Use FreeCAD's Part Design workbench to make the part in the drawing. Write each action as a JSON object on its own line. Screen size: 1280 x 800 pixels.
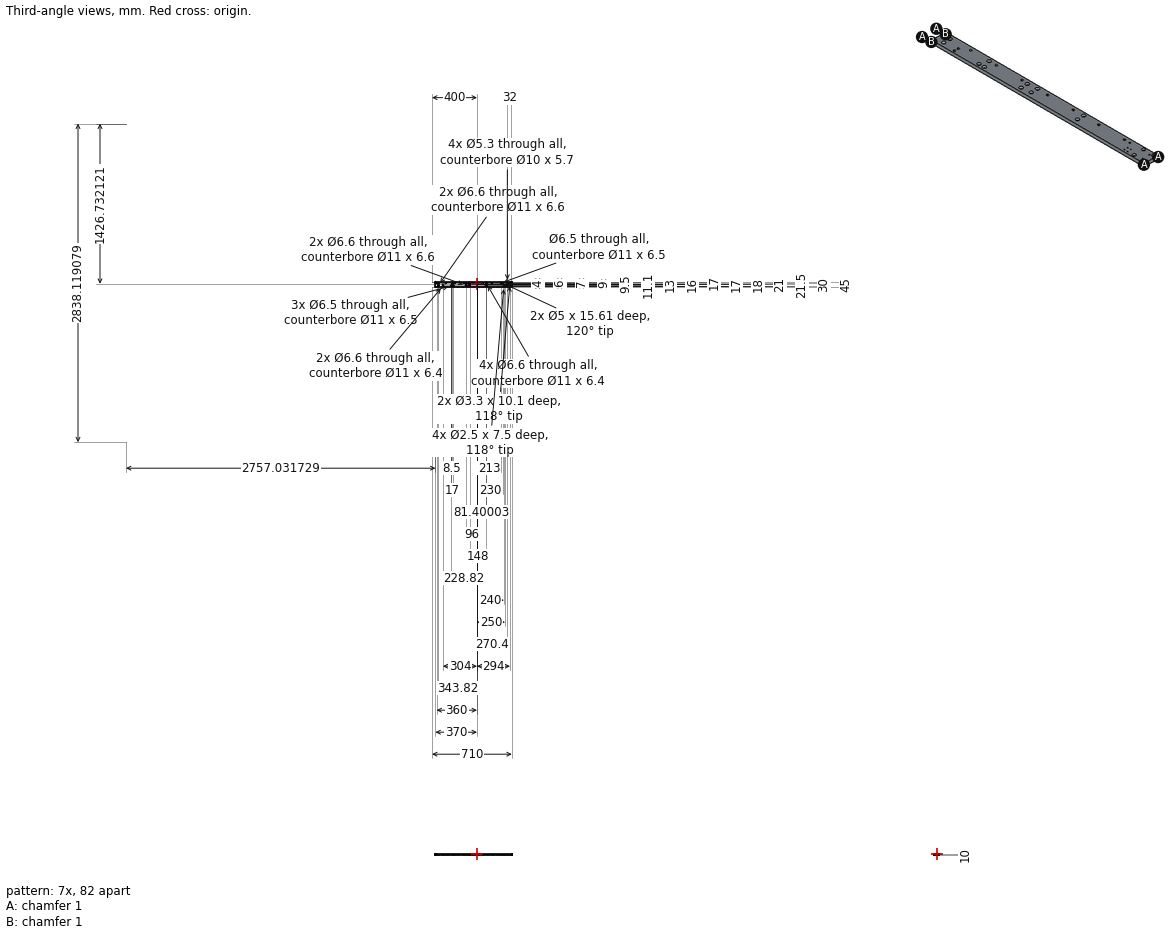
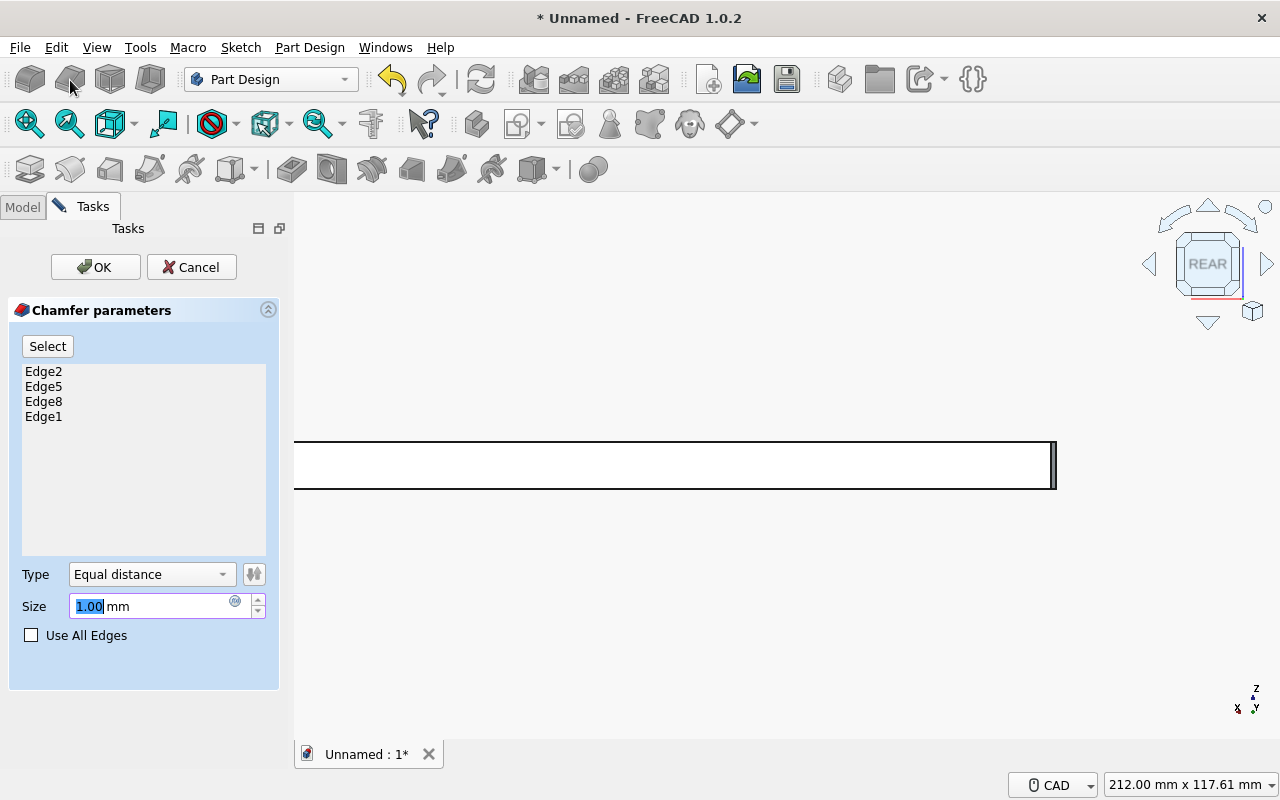
{"action": "type", "text": "1"}
{"action": "key", "text": "Tab"}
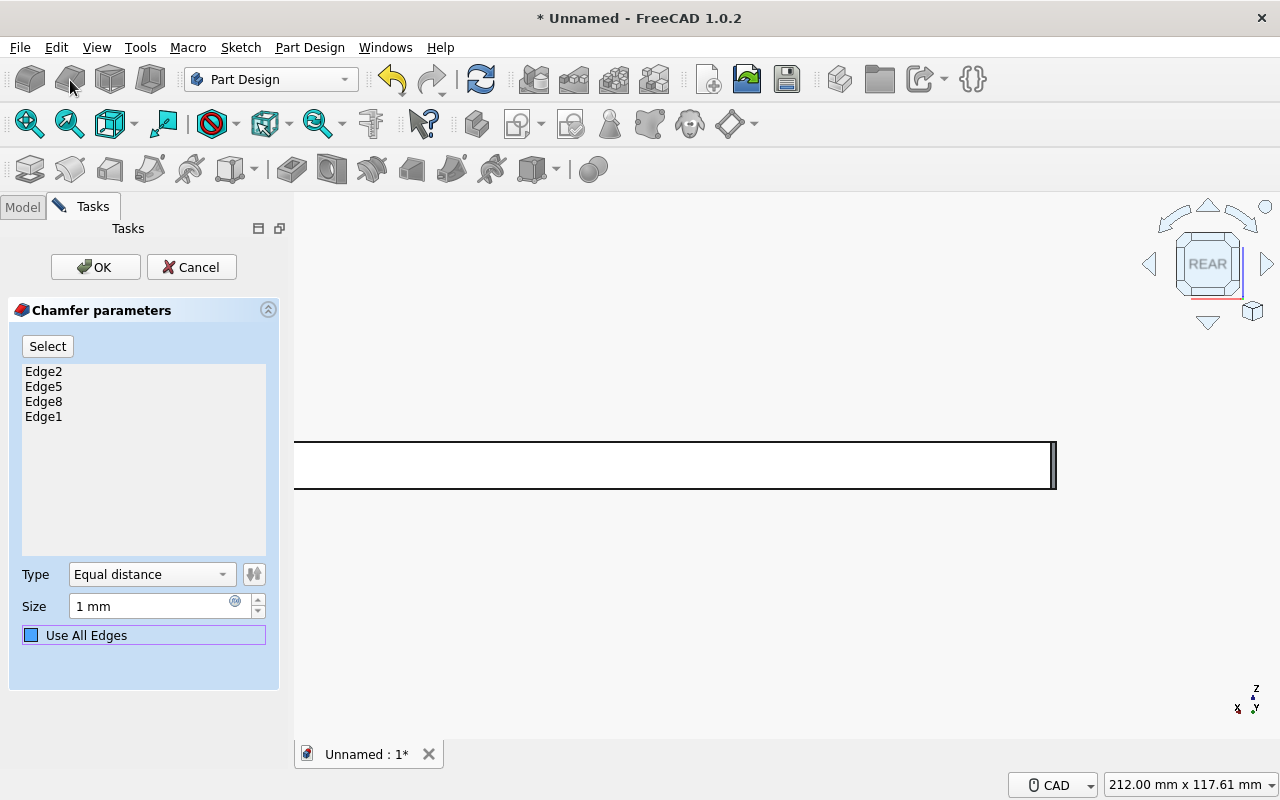
{"action": "left_click", "coordinate": [96, 267]}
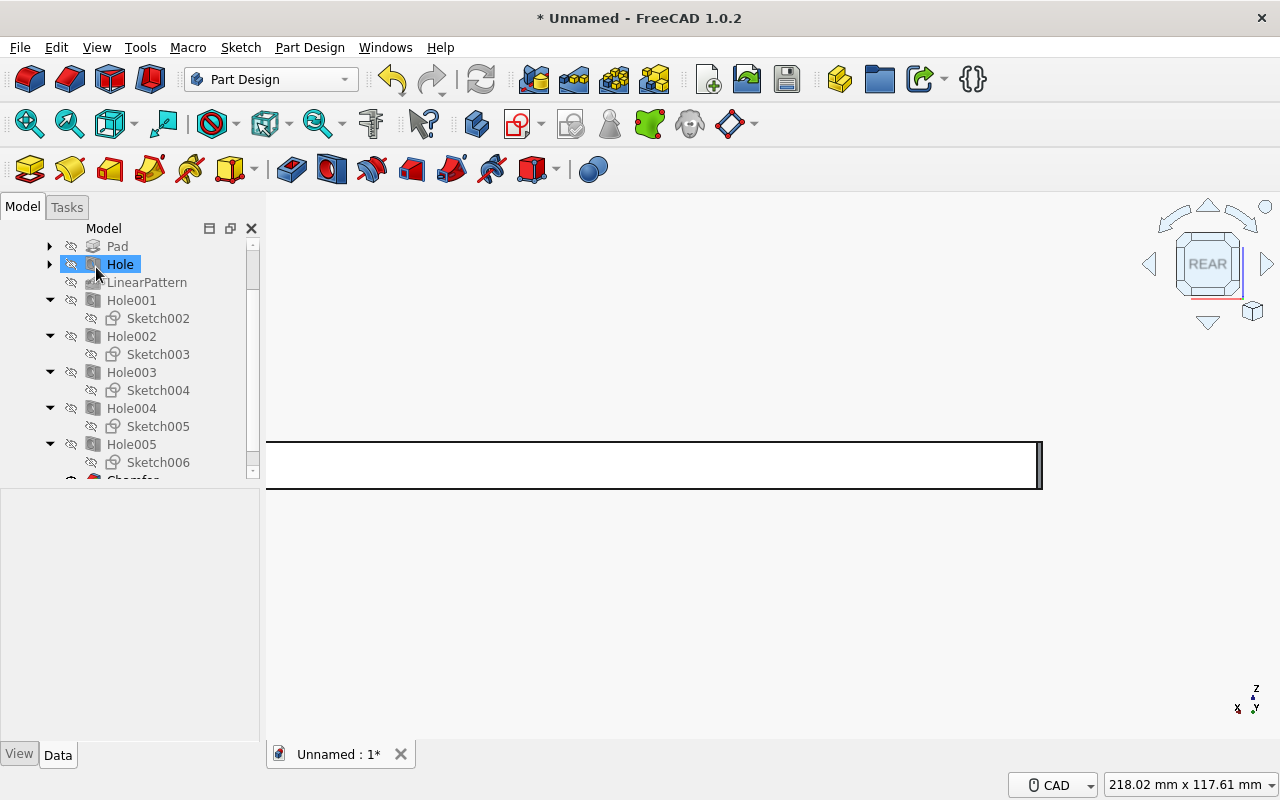
{"action": "left_click", "coordinate": [30, 124]}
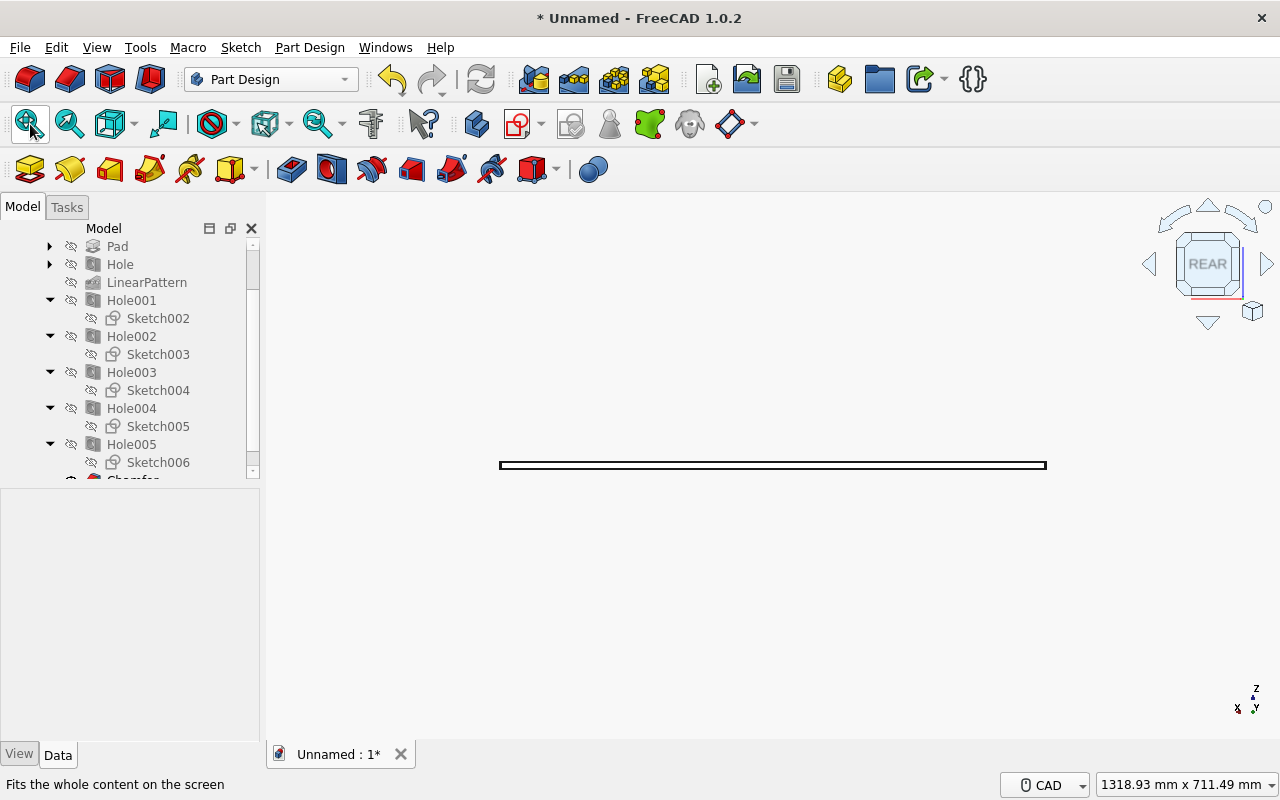
{"action": "left_click", "coordinate": [518, 124]}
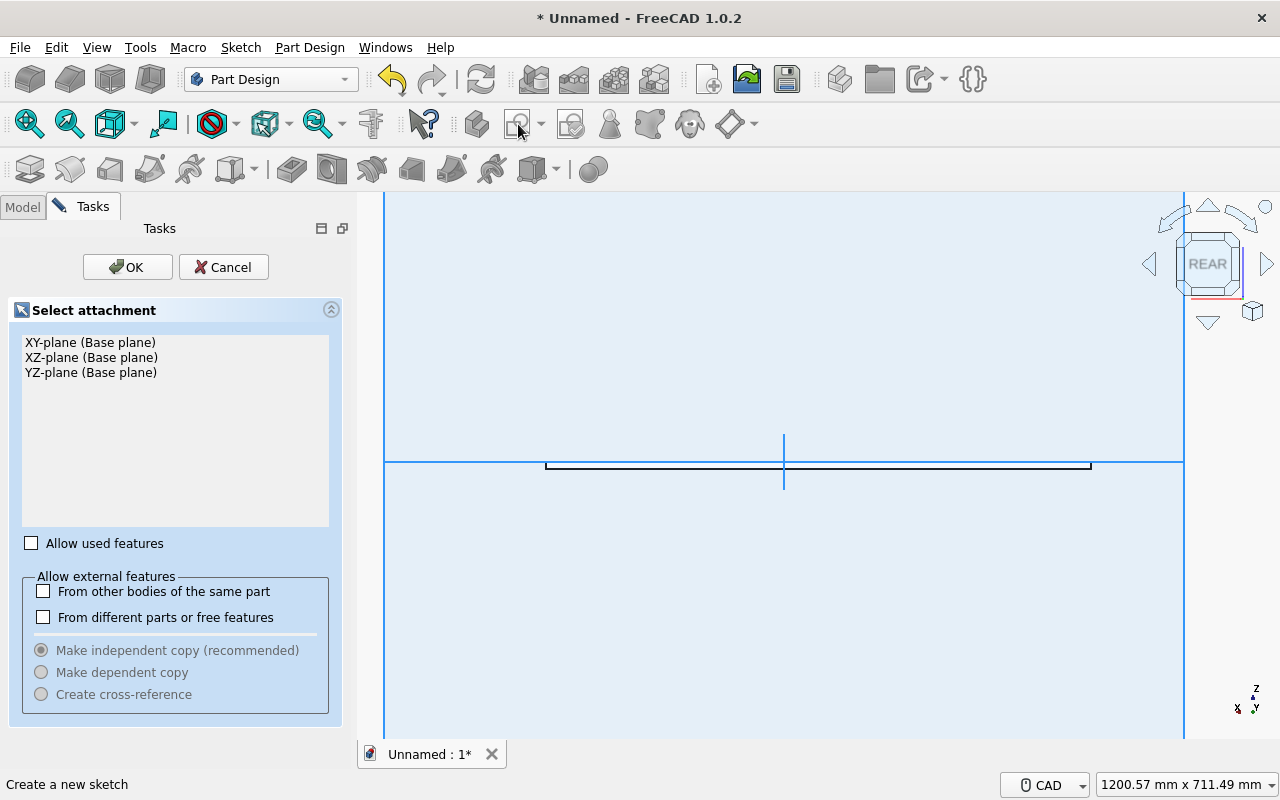
{"action": "left_click", "coordinate": [82, 342]}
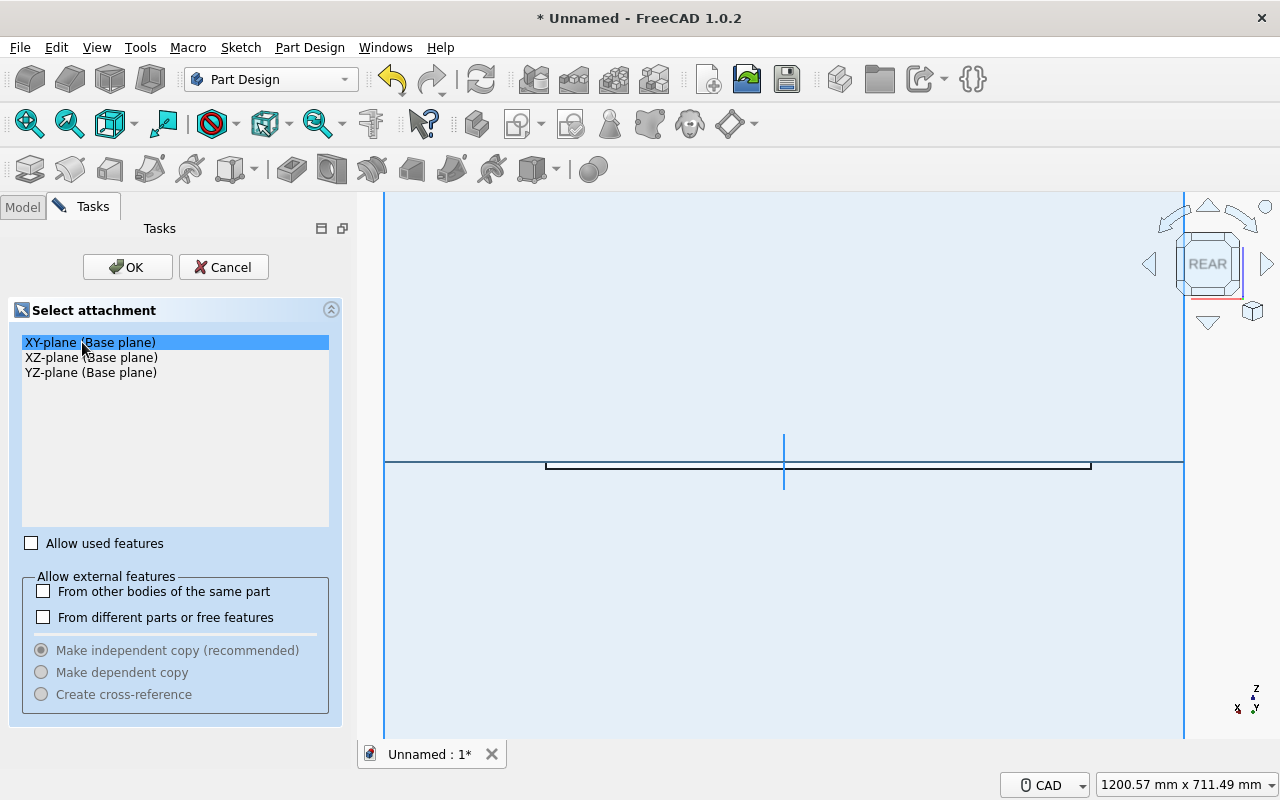
{"action": "left_click", "coordinate": [128, 267]}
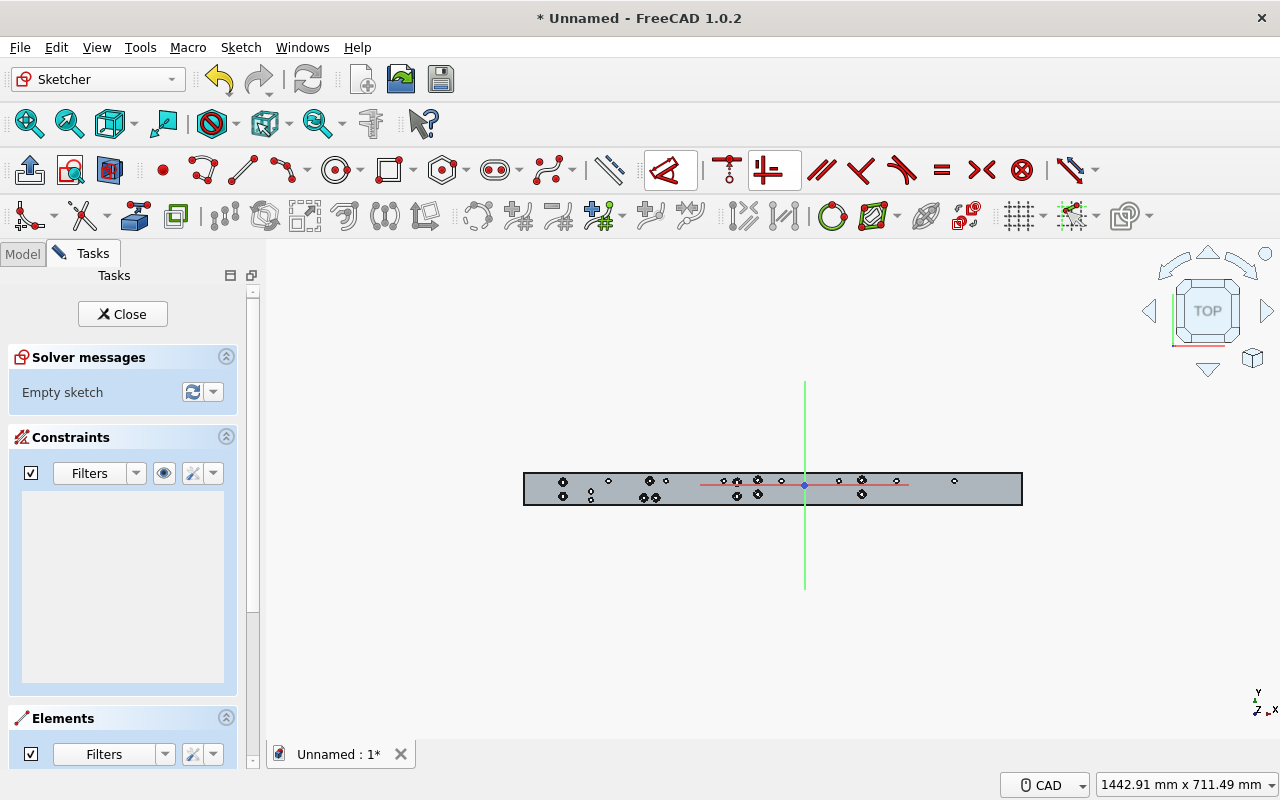
{"action": "scroll", "coordinate": [870, 468], "scroll_direction": "up", "scroll_amount": 2}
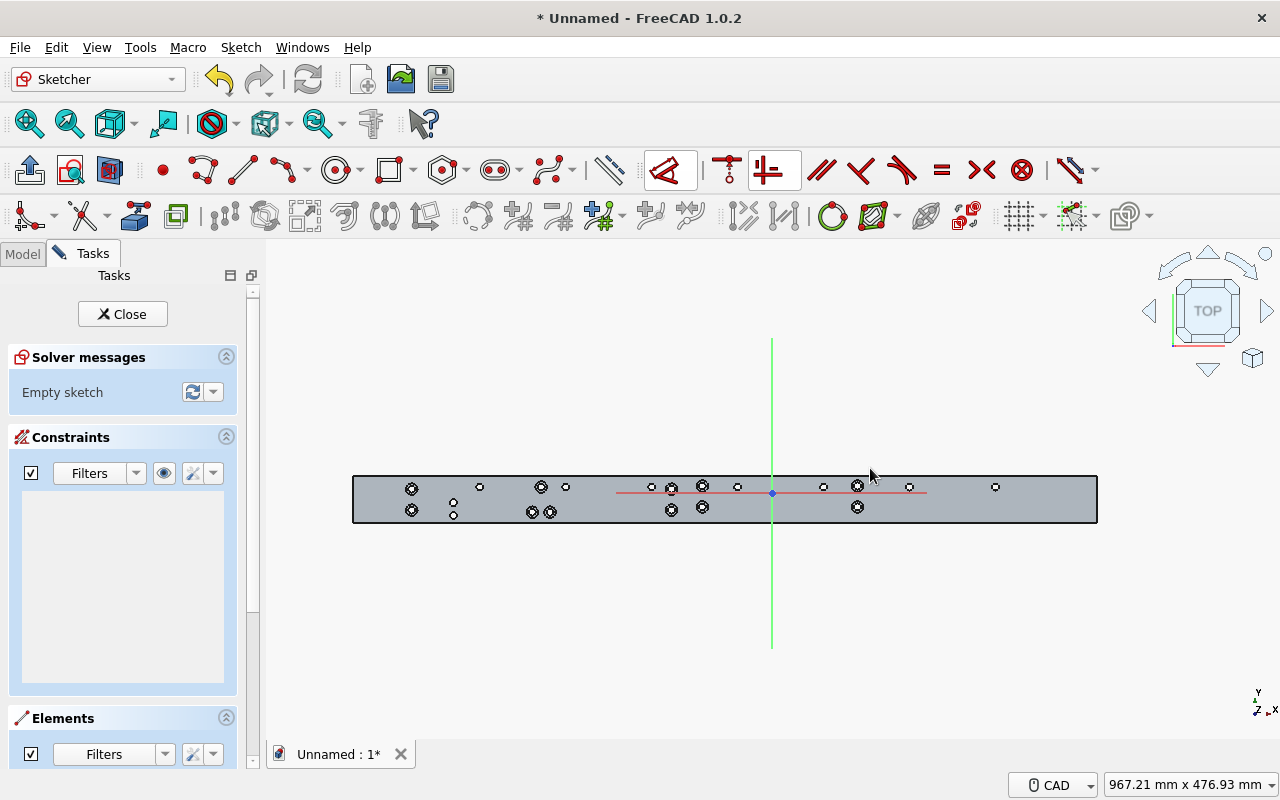
{"action": "left_click", "coordinate": [336, 170]}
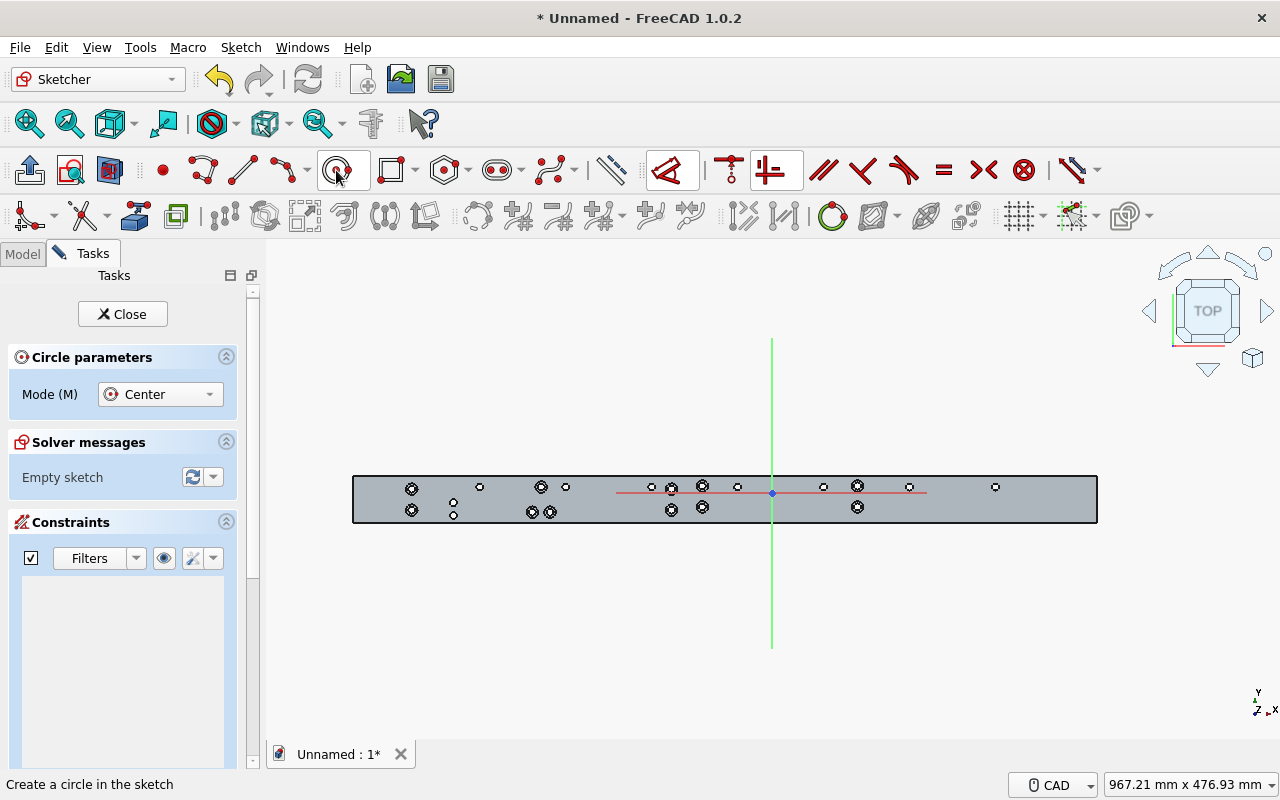
{"action": "scroll", "coordinate": [1013, 487], "scroll_direction": "up", "scroll_amount": 11}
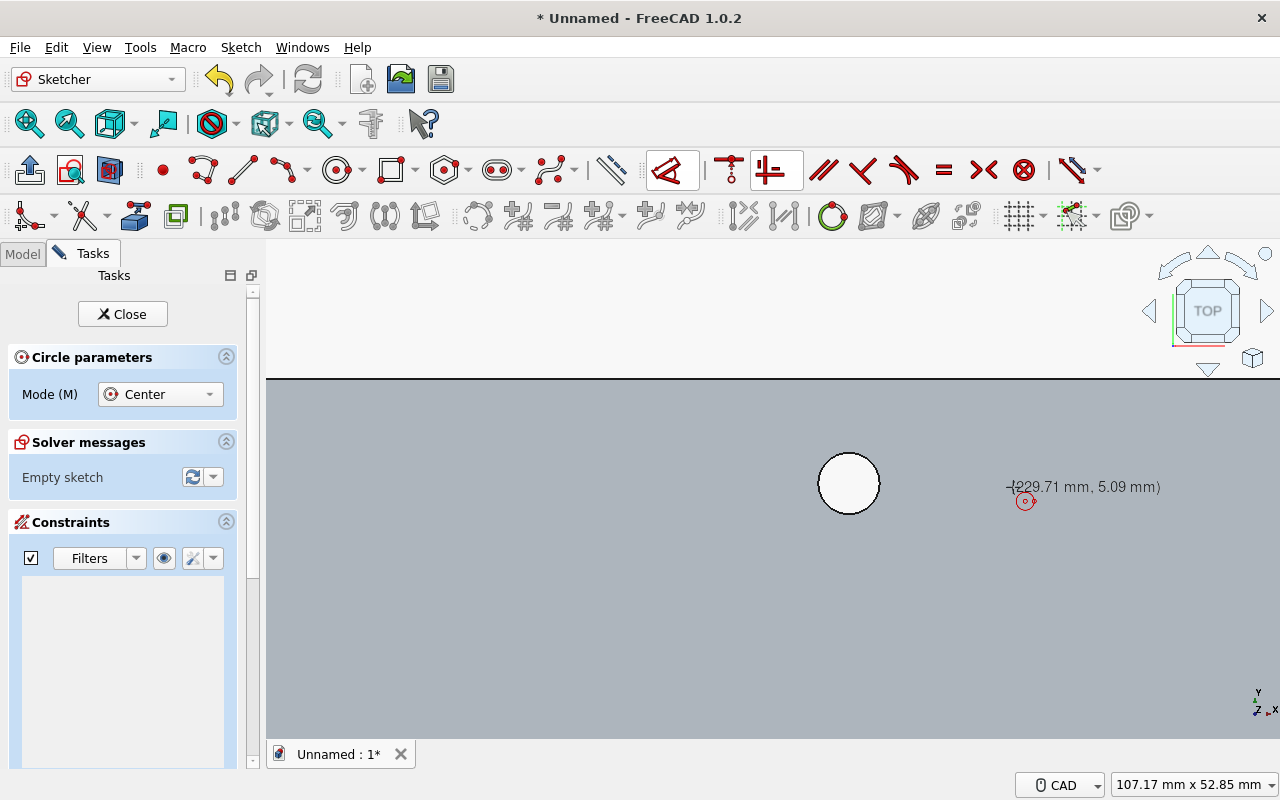
{"action": "scroll", "coordinate": [1014, 488], "scroll_direction": "down", "scroll_amount": 11}